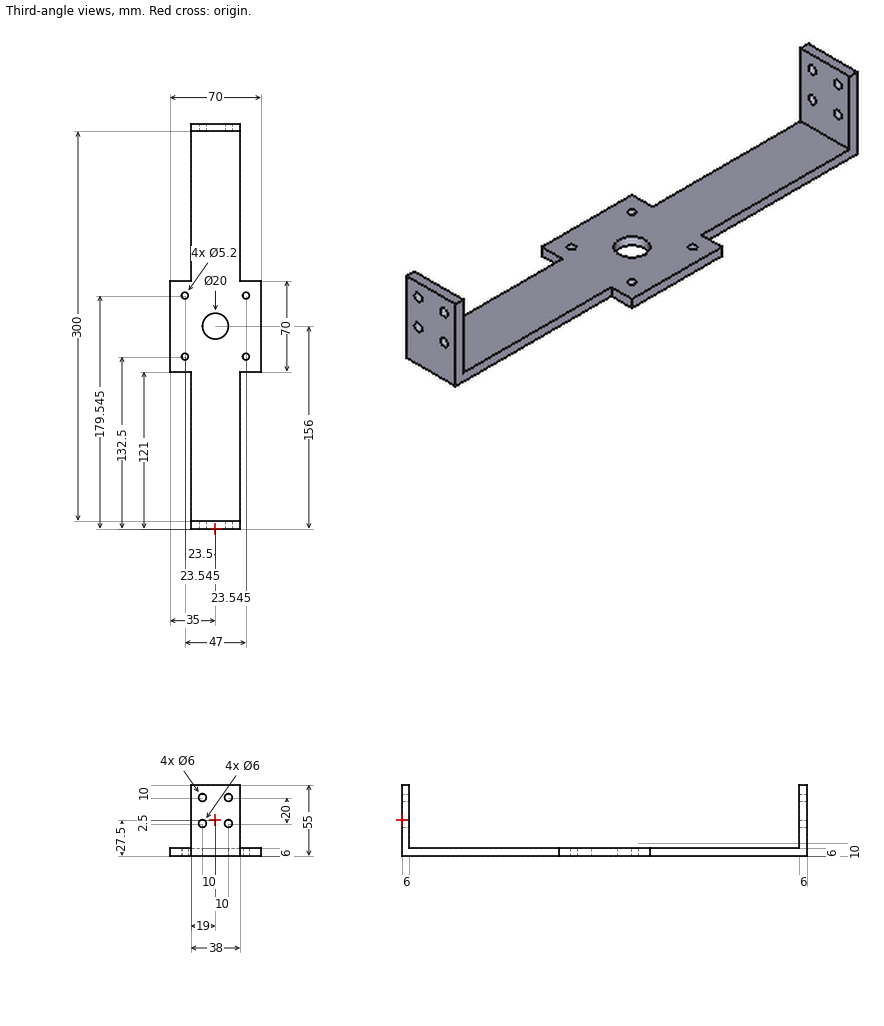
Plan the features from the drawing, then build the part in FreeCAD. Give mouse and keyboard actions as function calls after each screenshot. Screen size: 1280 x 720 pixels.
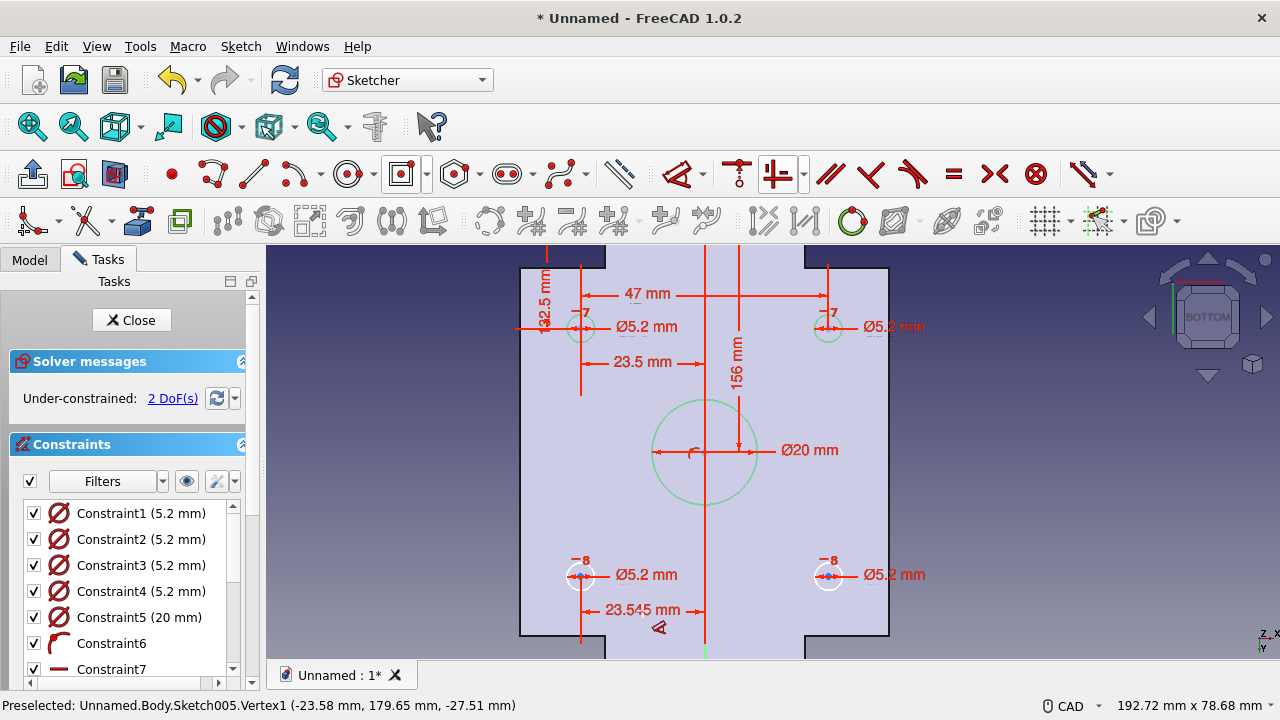
click(829, 577)
click(767, 611)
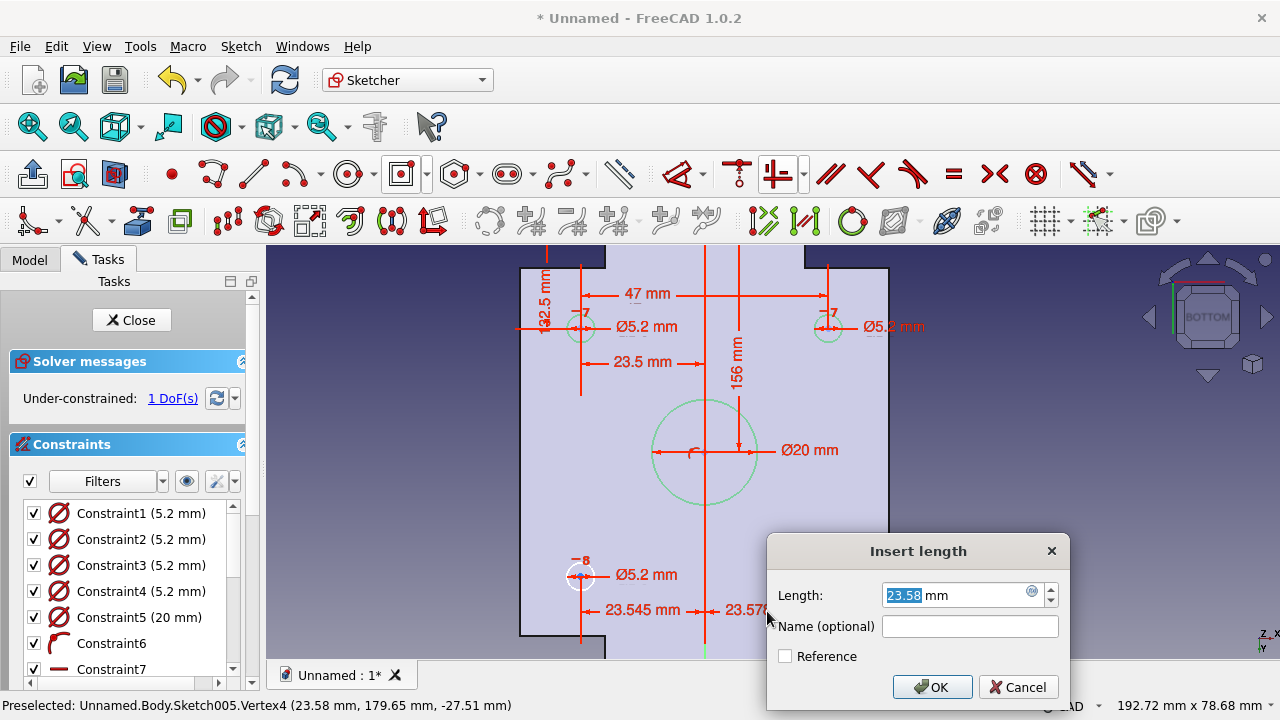
text(23.545)
key(Return)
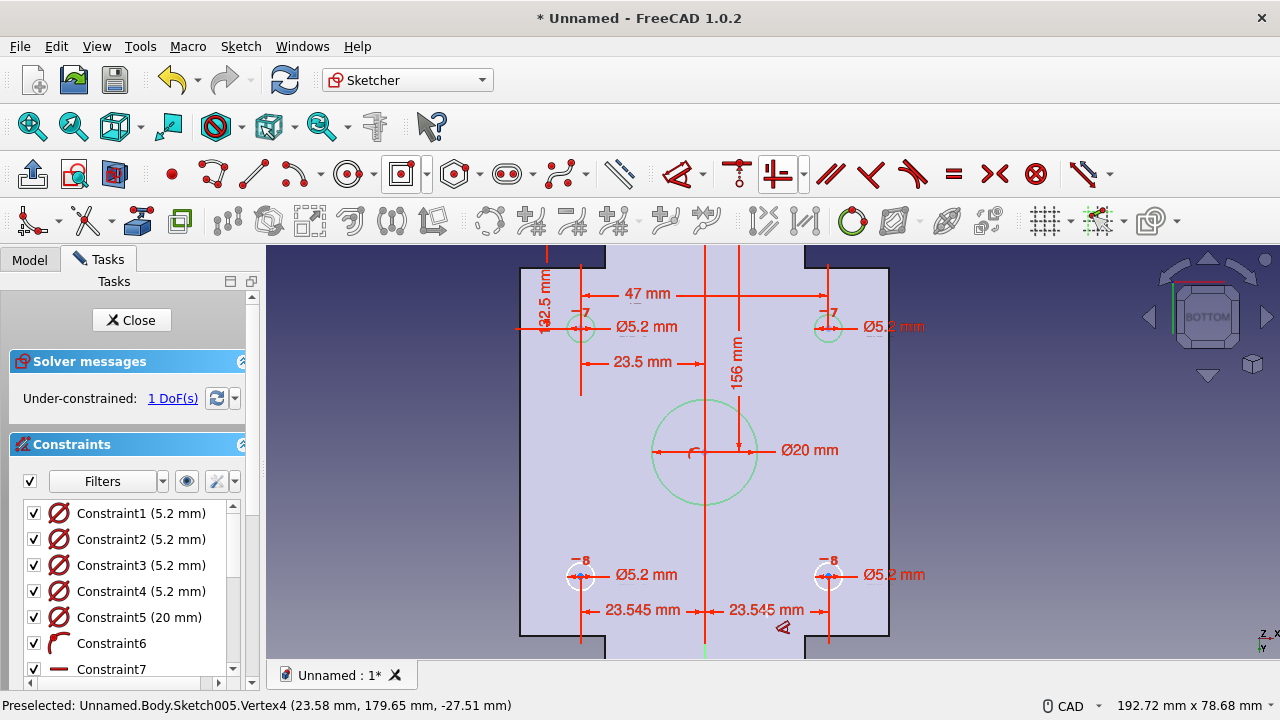
click(581, 577)
click(547, 425)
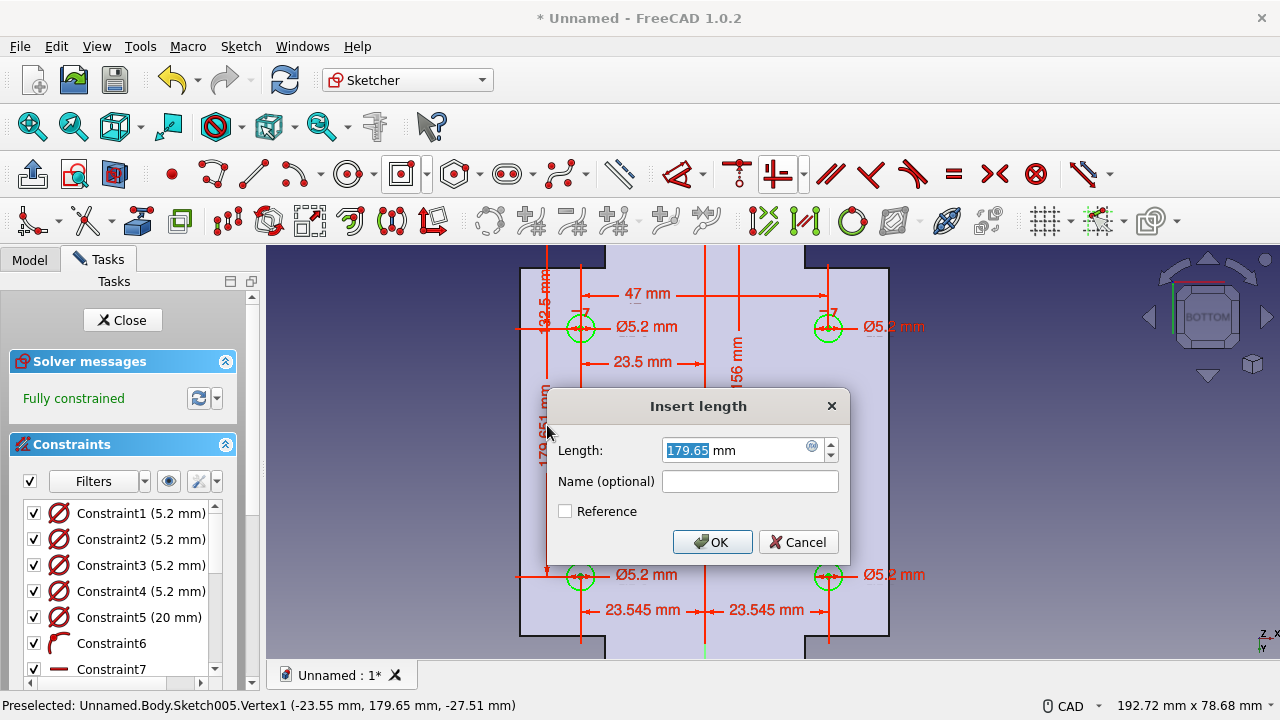
text(179.545)
key(Return)
key(Escape)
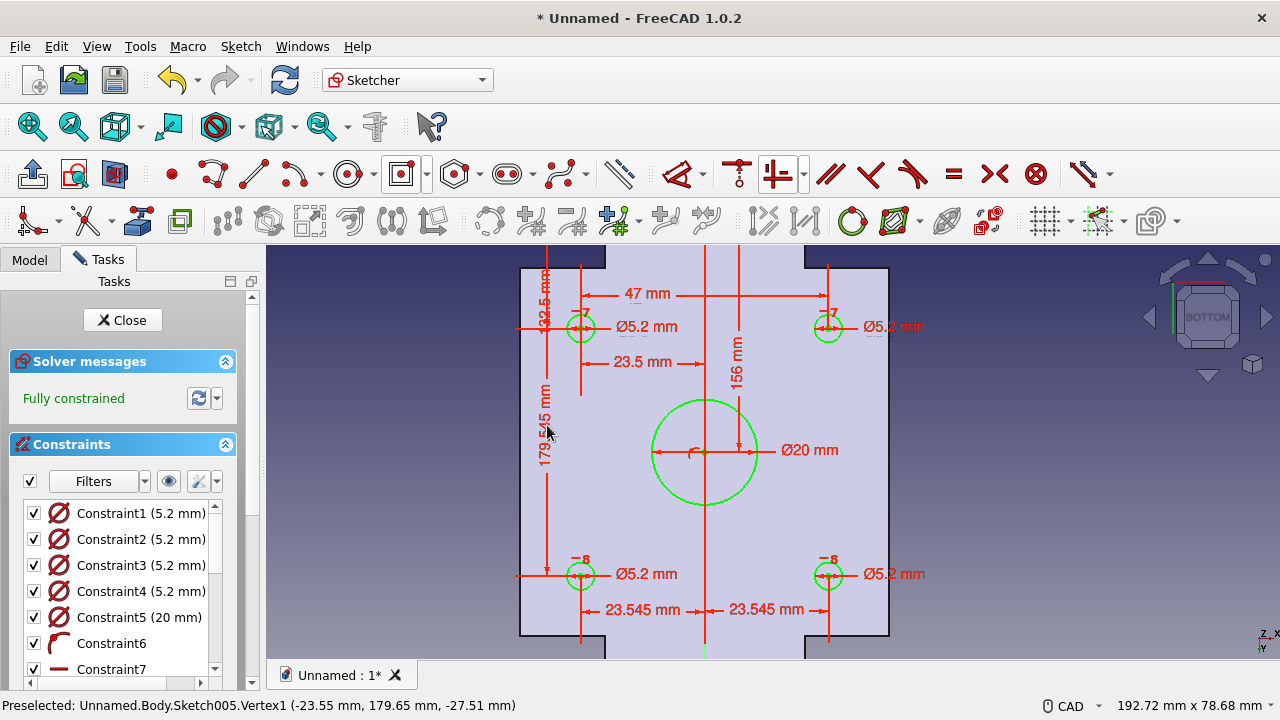
click(123, 320)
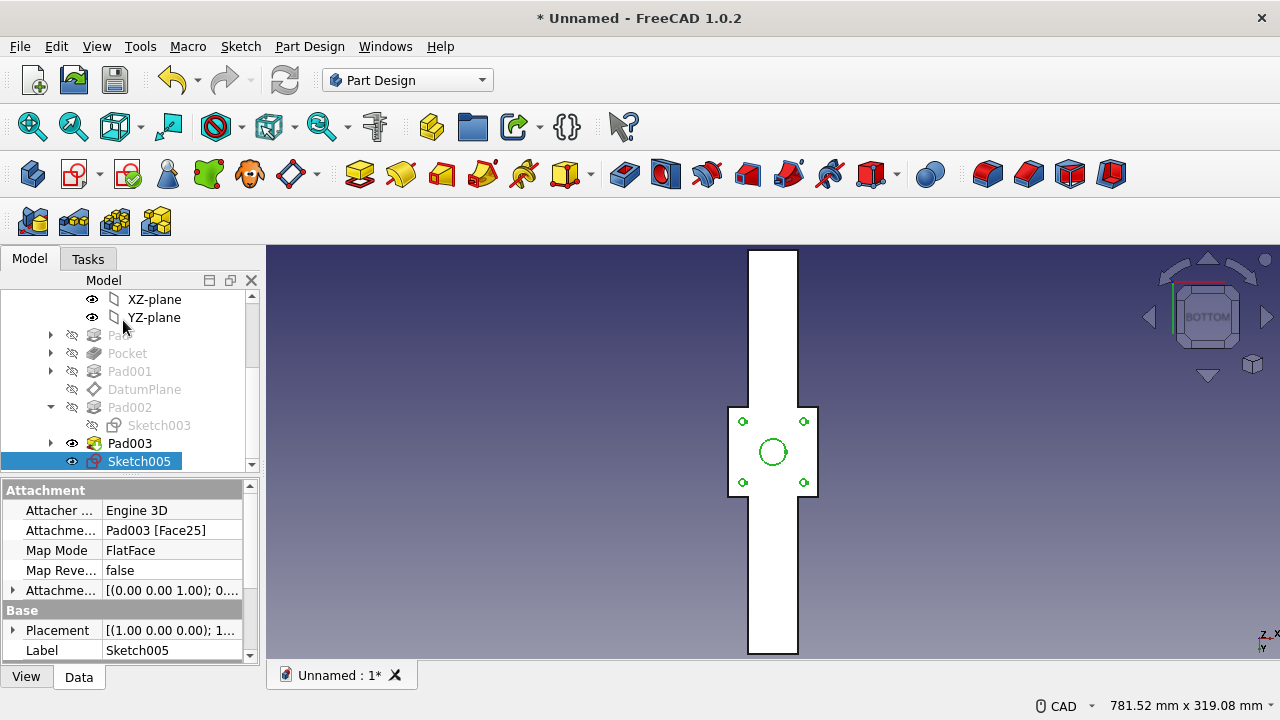
click(625, 174)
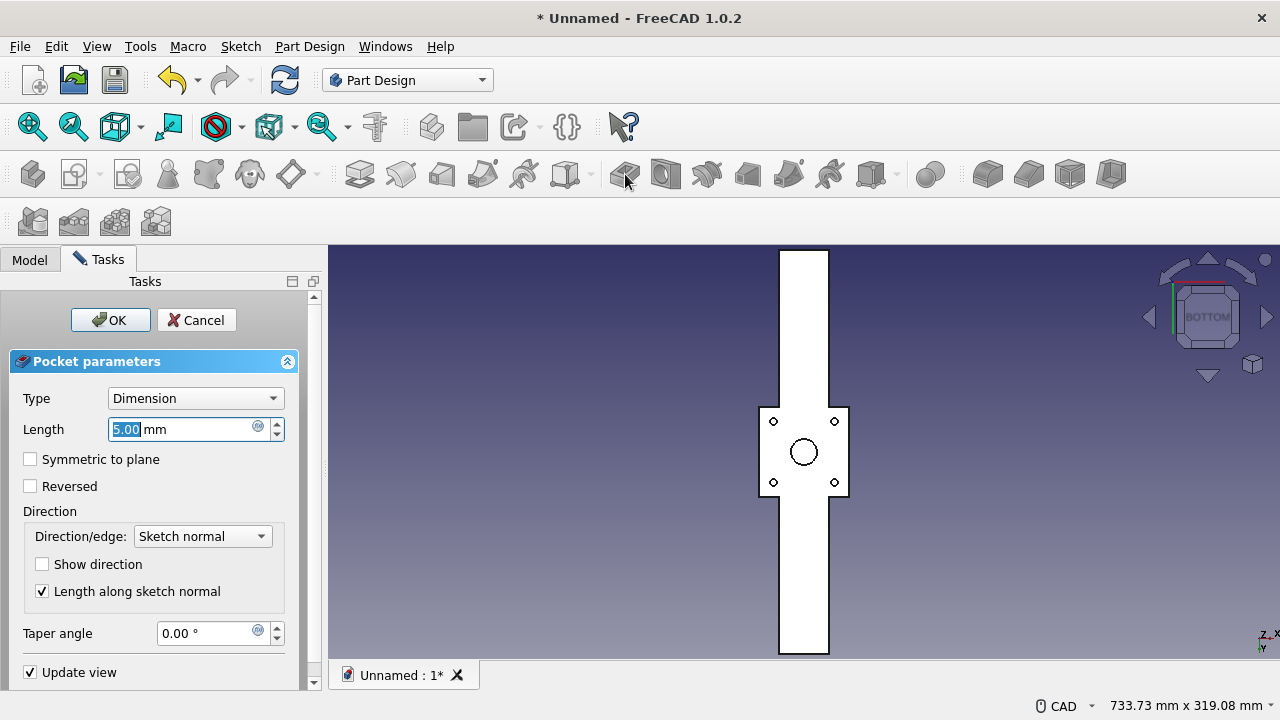
text(10)
key(Tab)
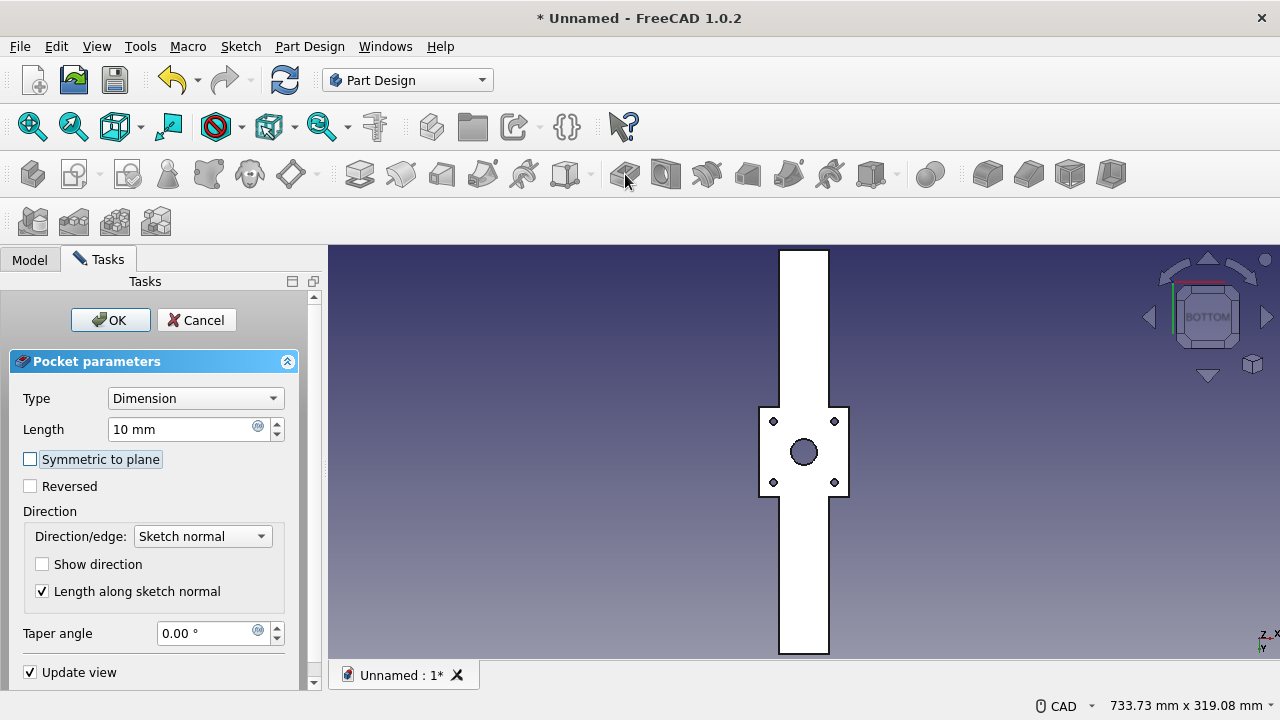
click(111, 320)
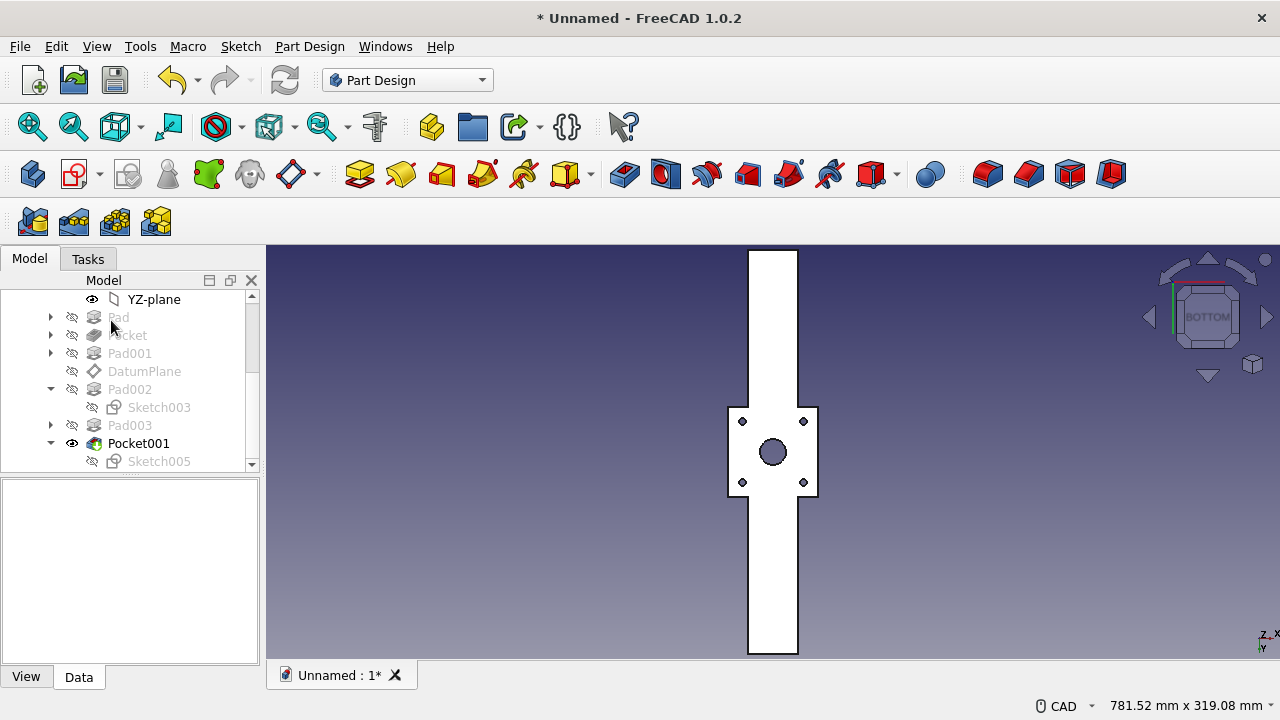
key(0)